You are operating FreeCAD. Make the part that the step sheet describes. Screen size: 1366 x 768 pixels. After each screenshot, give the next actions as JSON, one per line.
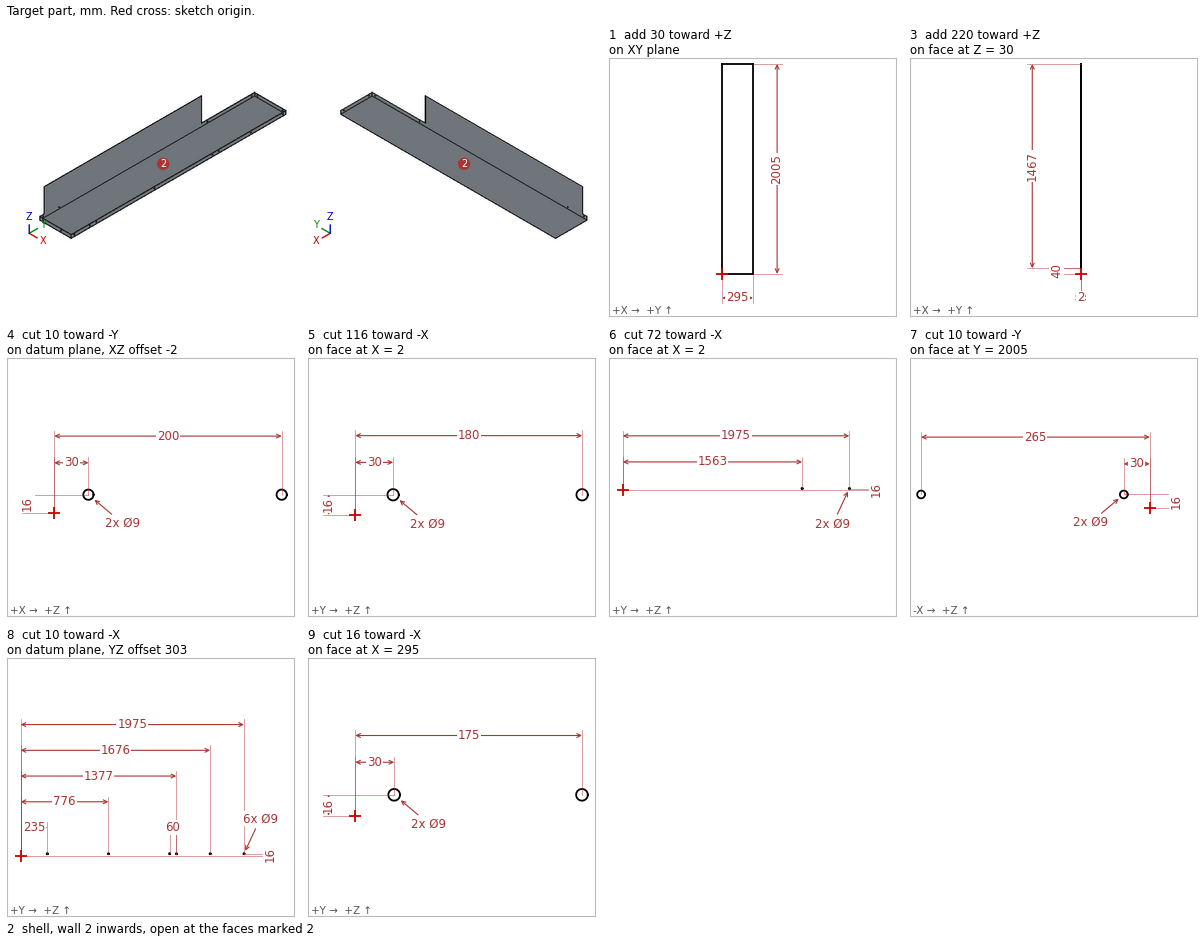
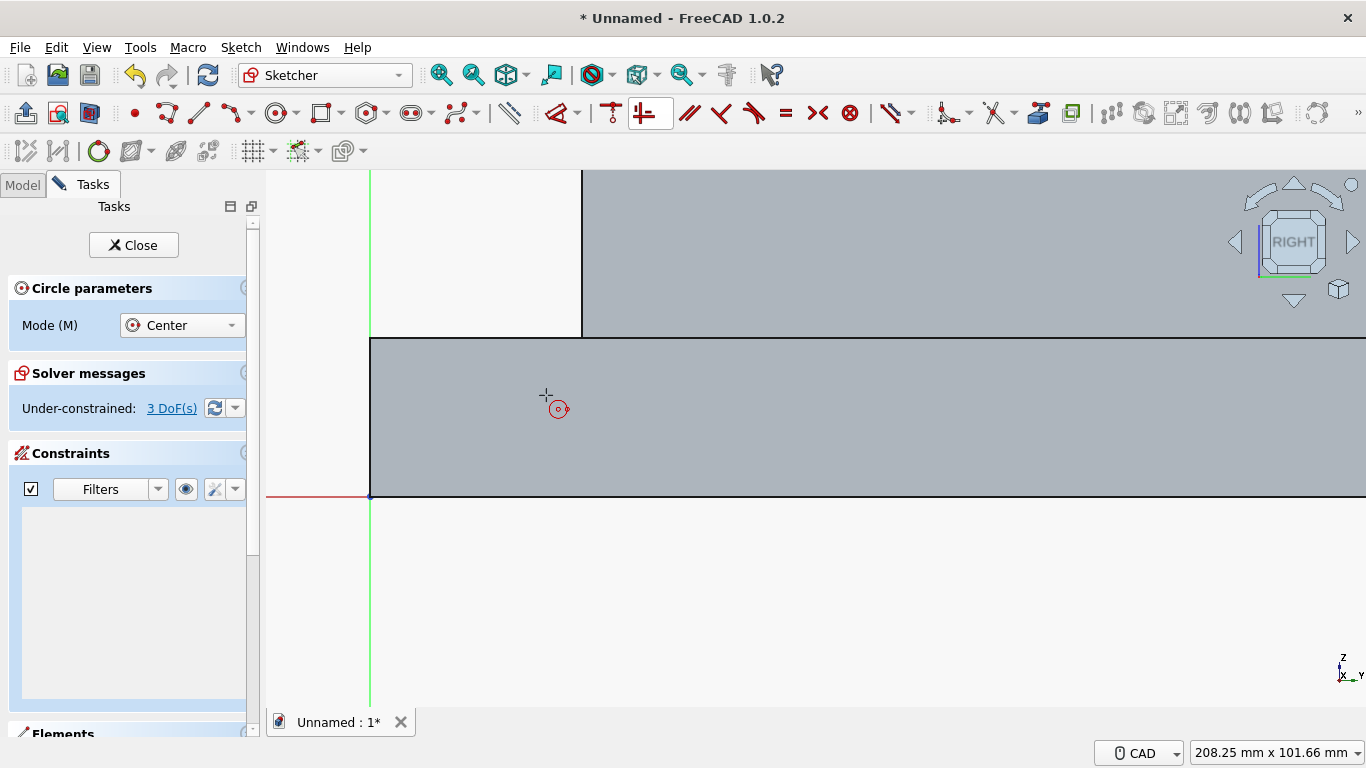
{"action": "scroll", "coordinate": [524, 430], "scroll_direction": "down", "scroll_amount": 2}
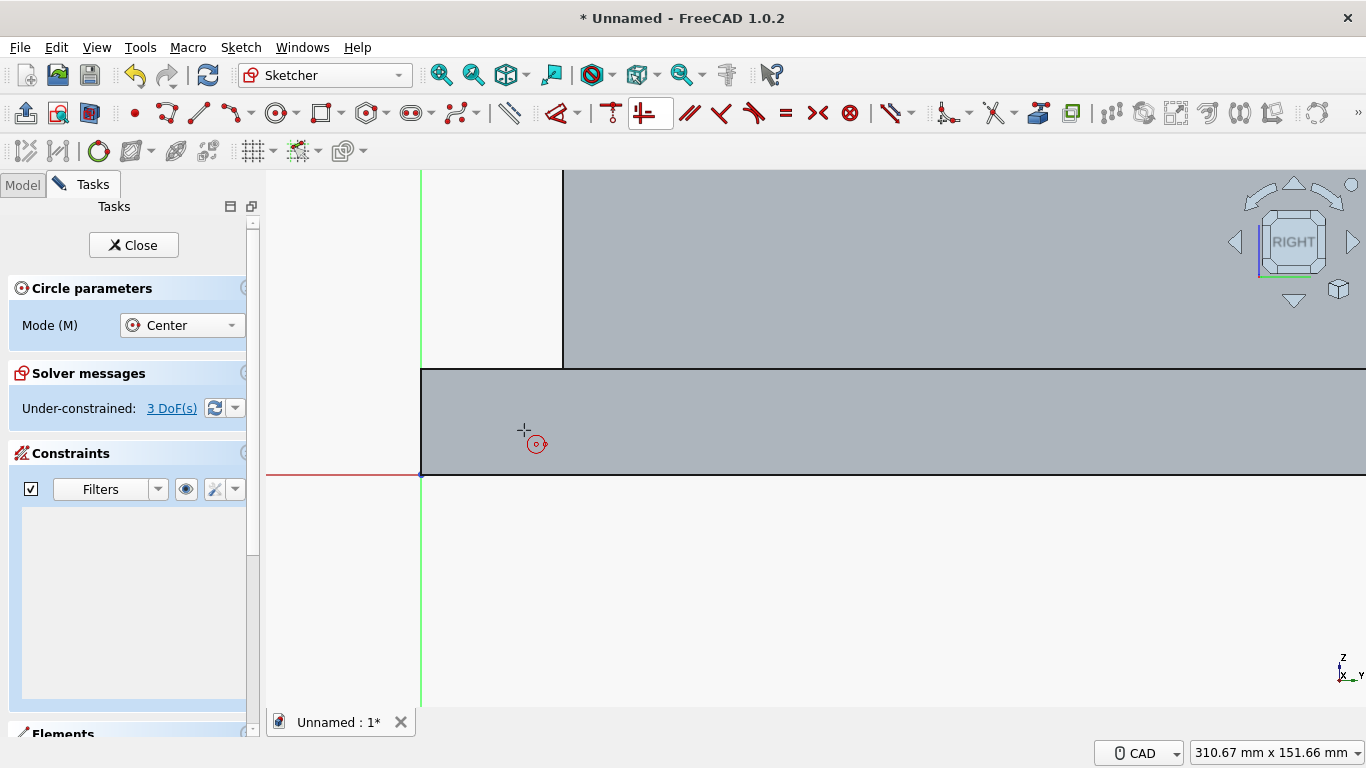
{"action": "scroll", "coordinate": [1058, 418], "scroll_direction": "up", "scroll_amount": 2}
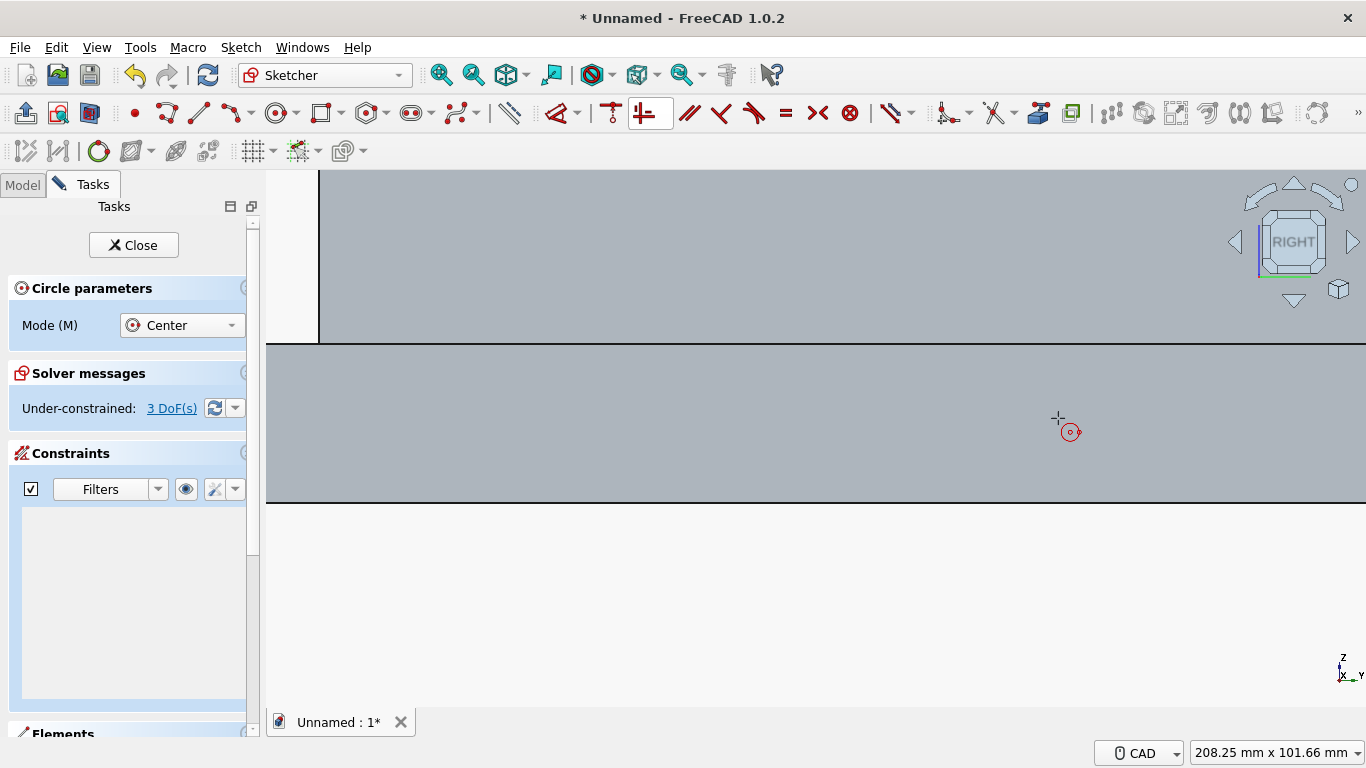
{"action": "left_click", "coordinate": [1058, 418]}
{"action": "left_click", "coordinate": [1075, 401]}
{"action": "key", "text": "Escape"}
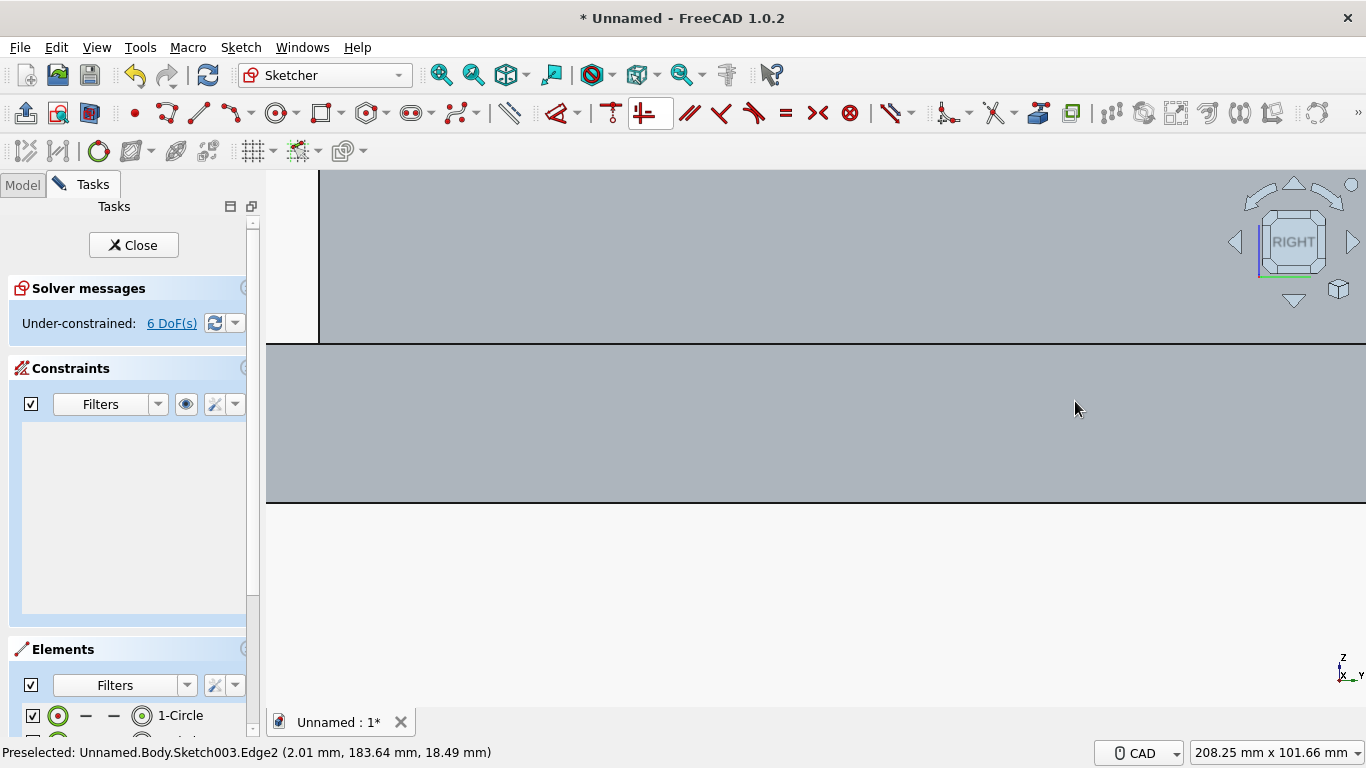
{"action": "scroll", "coordinate": [1058, 418], "scroll_direction": "down", "scroll_amount": 2}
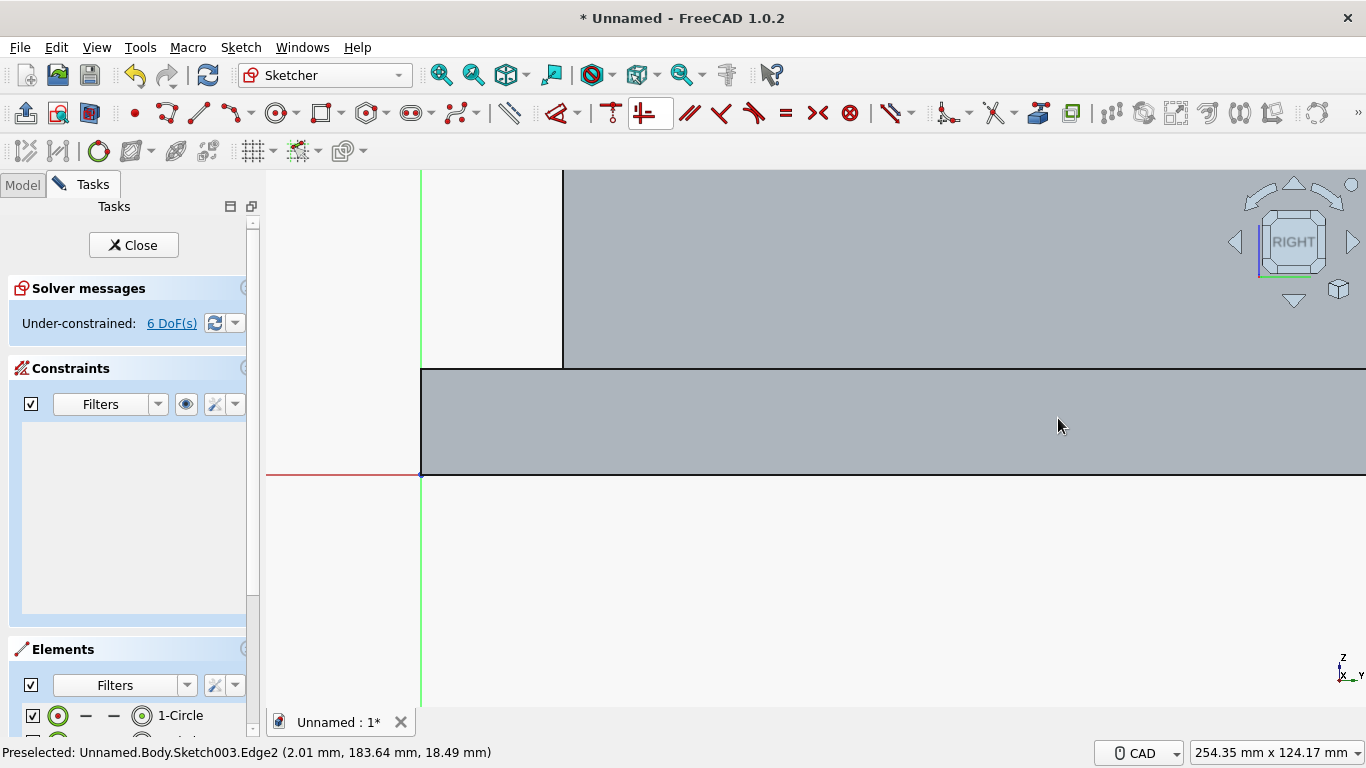
{"action": "left_click", "coordinate": [539, 407]}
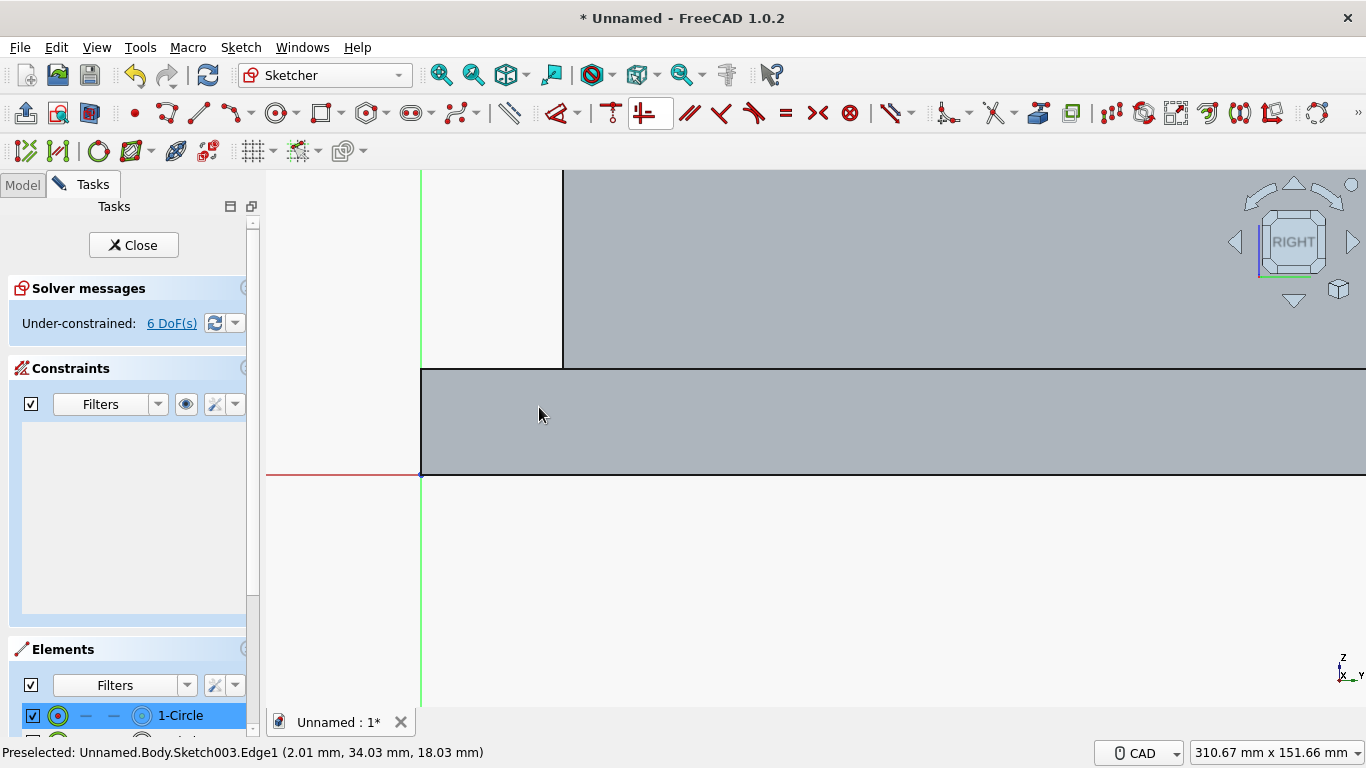
{"action": "left_click", "coordinate": [1070, 407]}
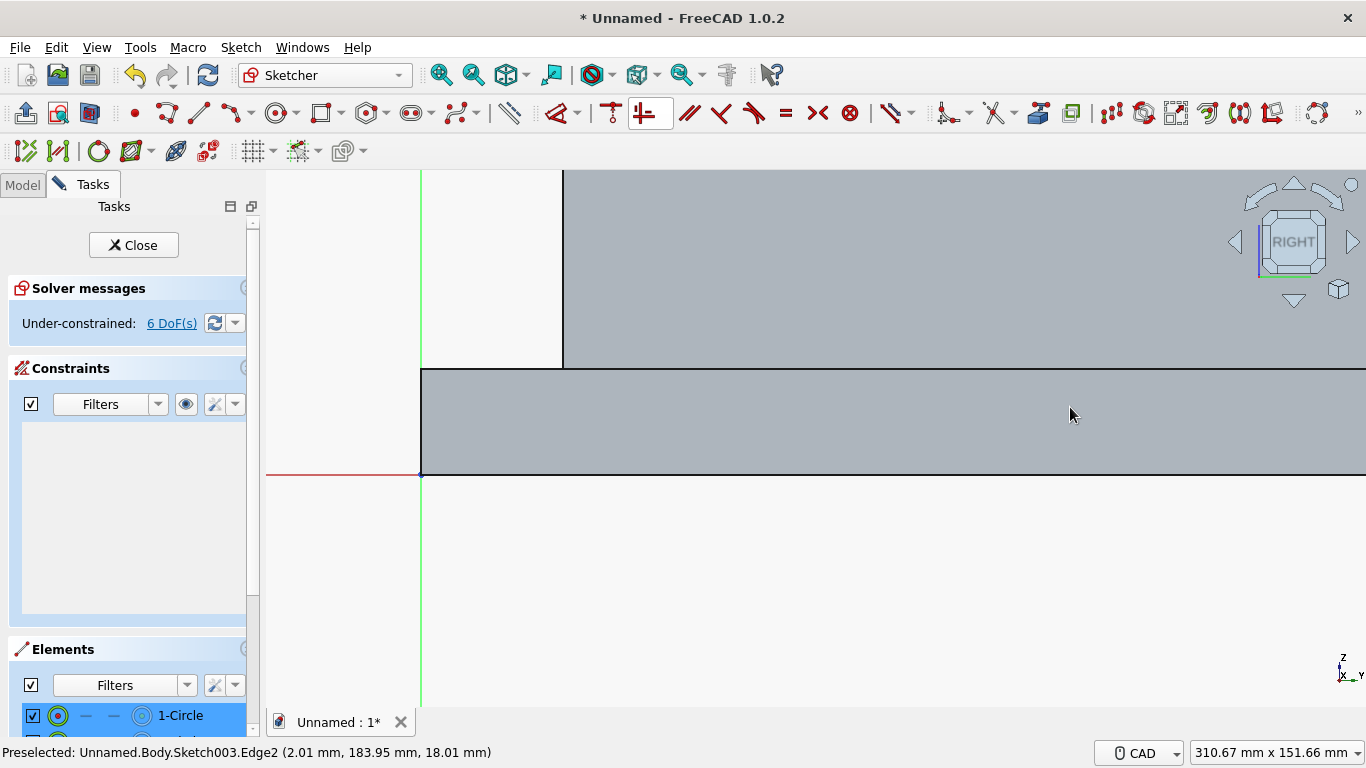
{"action": "left_click", "coordinate": [786, 114]}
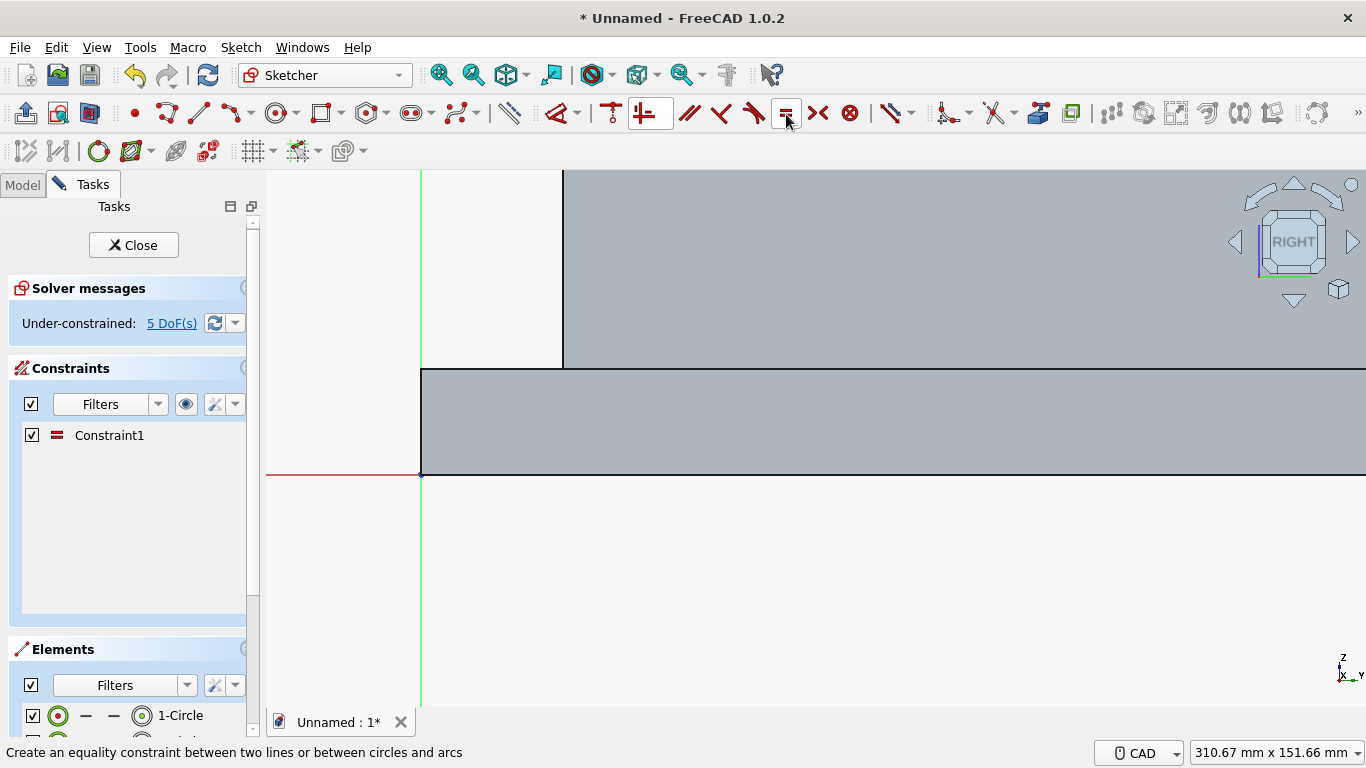
{"action": "left_click", "coordinate": [527, 419]}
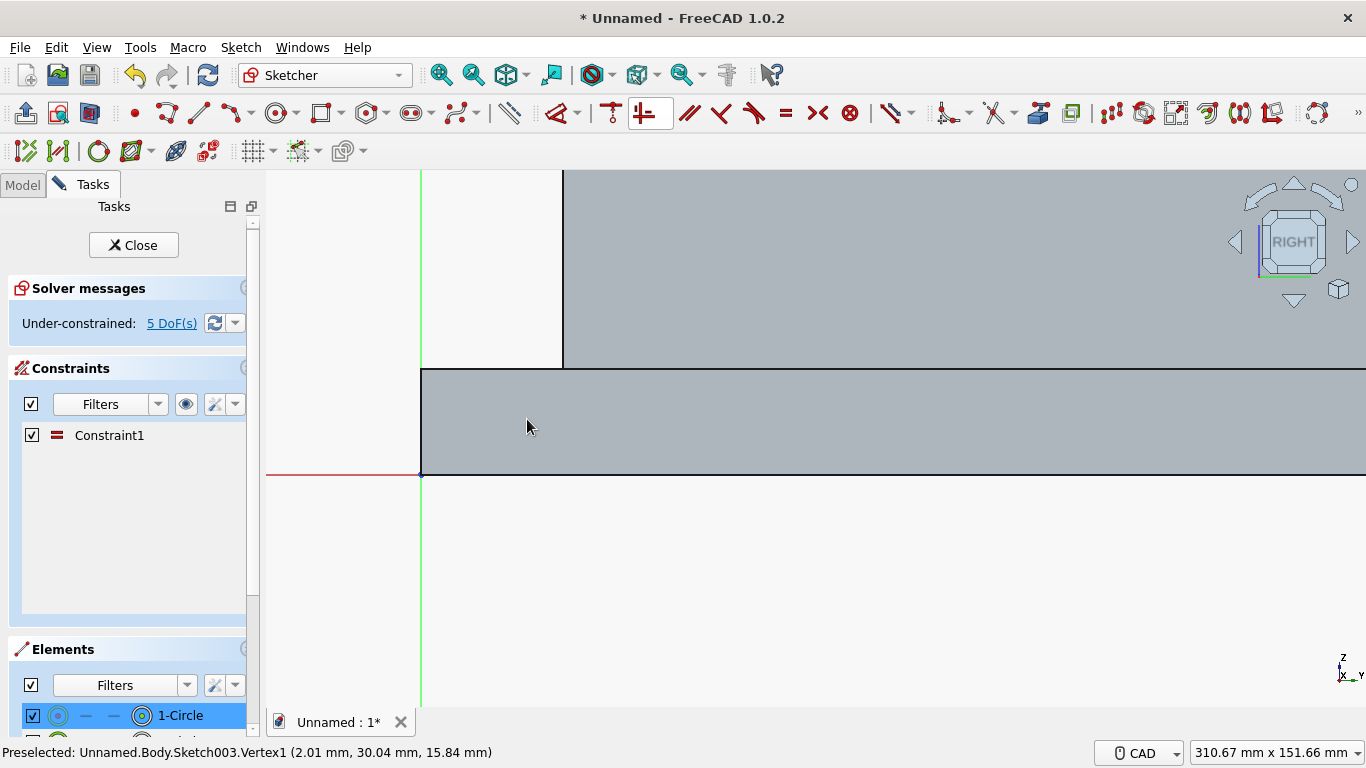
{"action": "left_click", "coordinate": [1058, 419]}